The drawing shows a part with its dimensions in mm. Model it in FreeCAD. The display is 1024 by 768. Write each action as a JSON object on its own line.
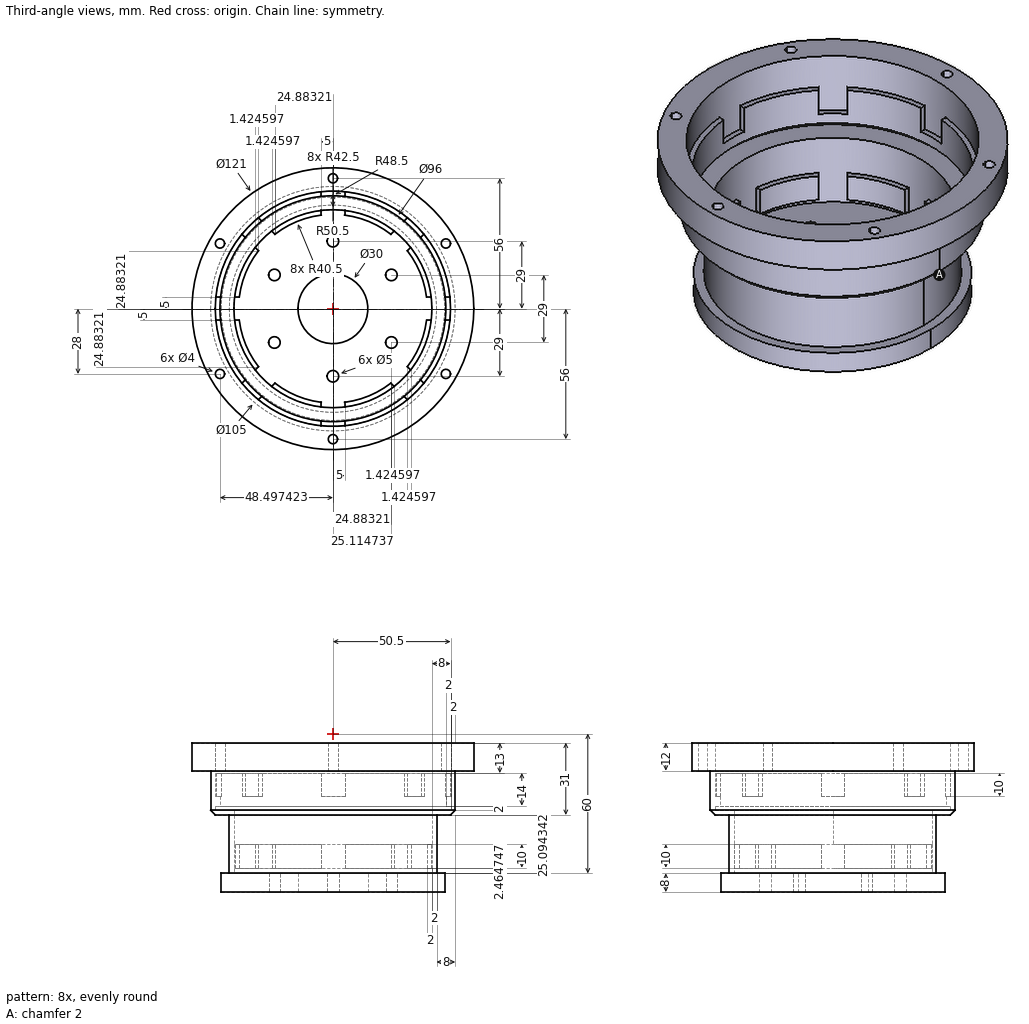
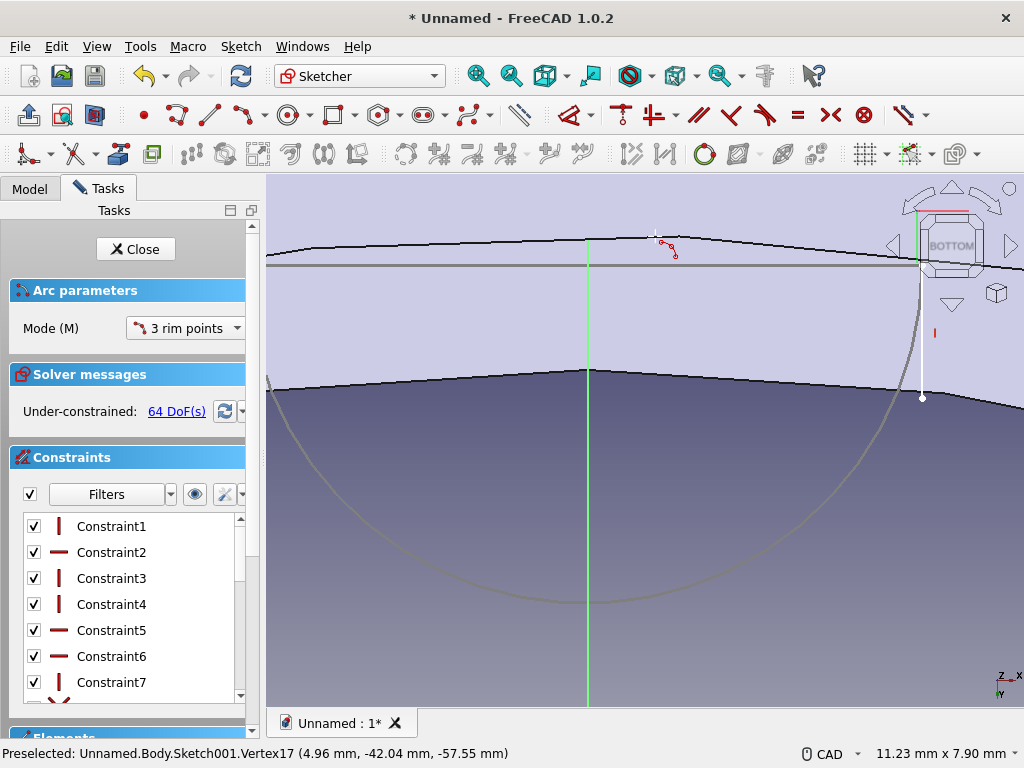
{"action": "left_click", "coordinate": [655, 236]}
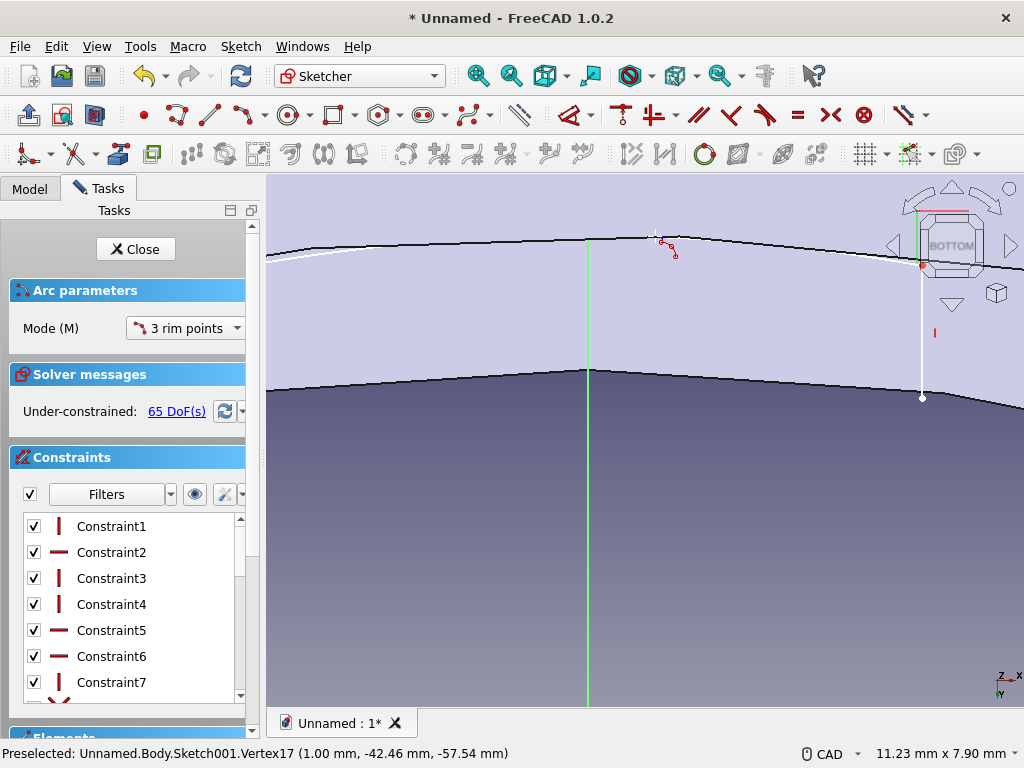
{"action": "scroll", "coordinate": [576, 268], "scroll_direction": "down", "scroll_amount": 14}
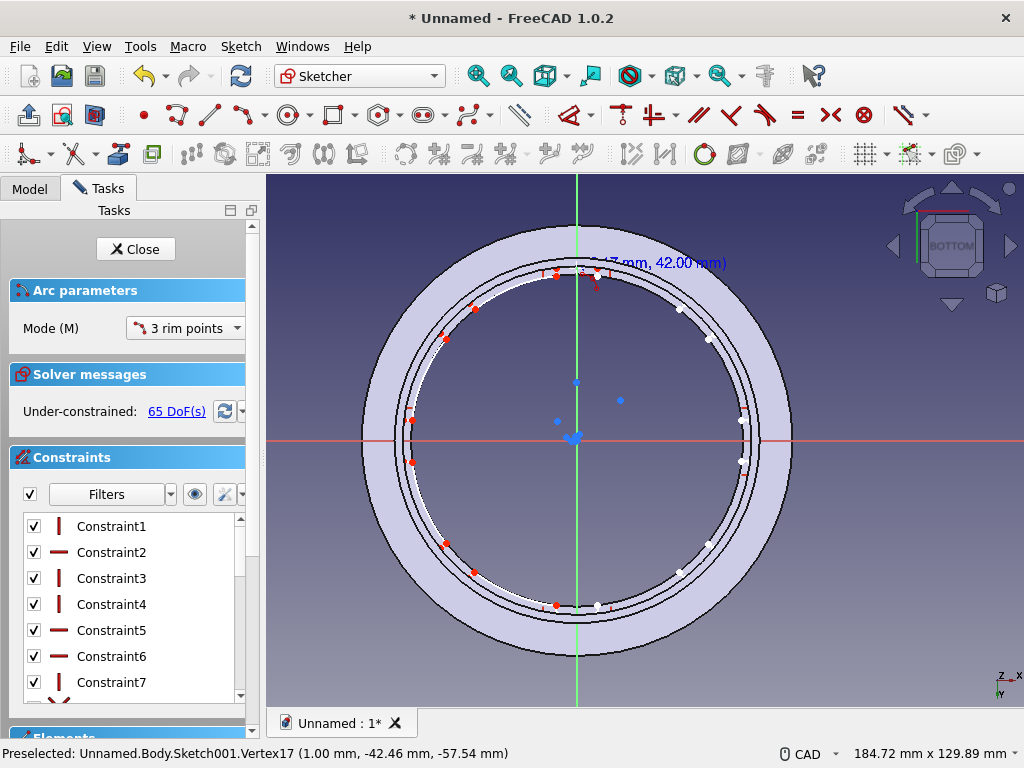
{"action": "scroll", "coordinate": [598, 276], "scroll_direction": "up", "scroll_amount": 7}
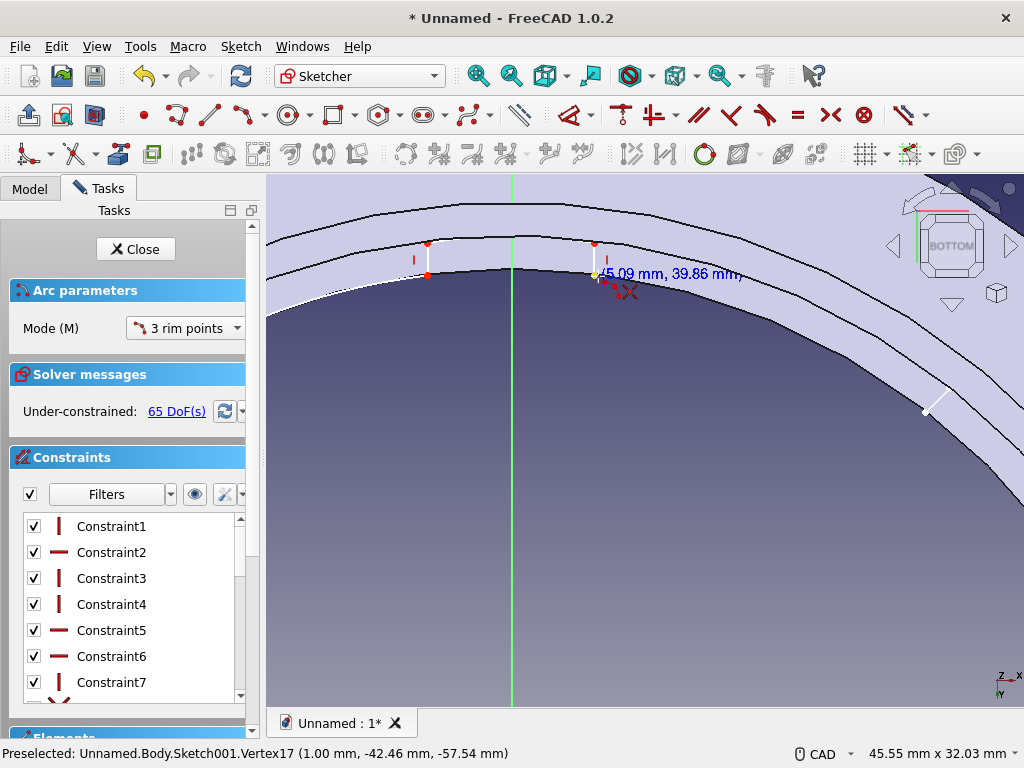
{"action": "left_click", "coordinate": [594, 276]}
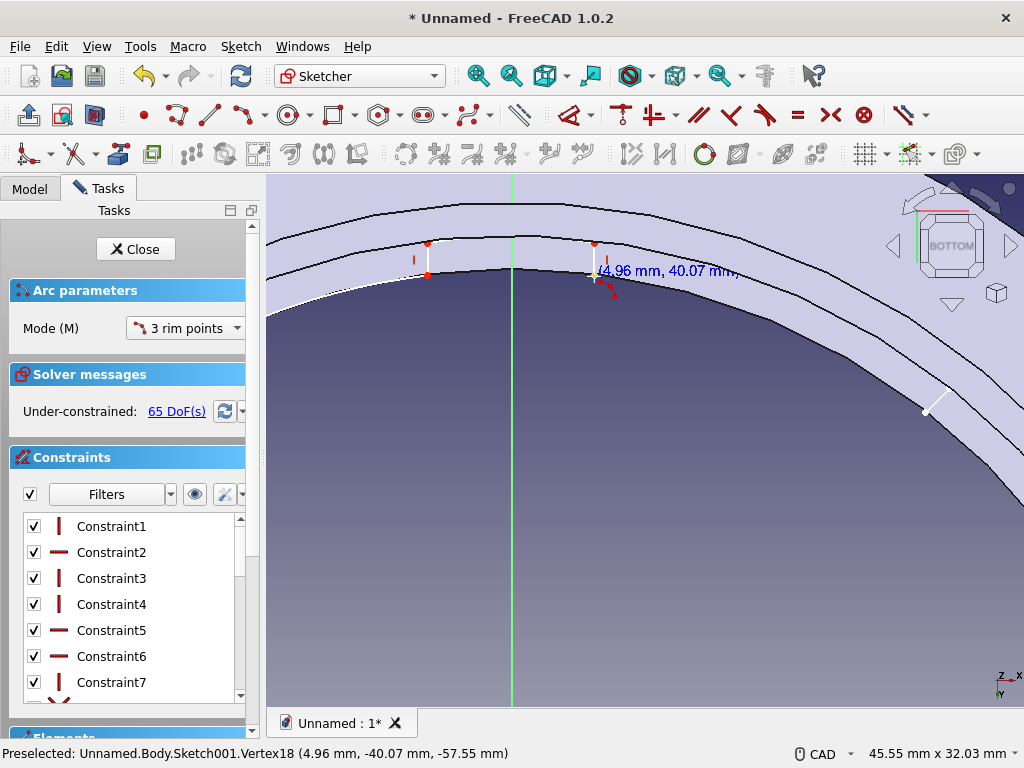
{"action": "scroll", "coordinate": [598, 276], "scroll_direction": "down", "scroll_amount": 7}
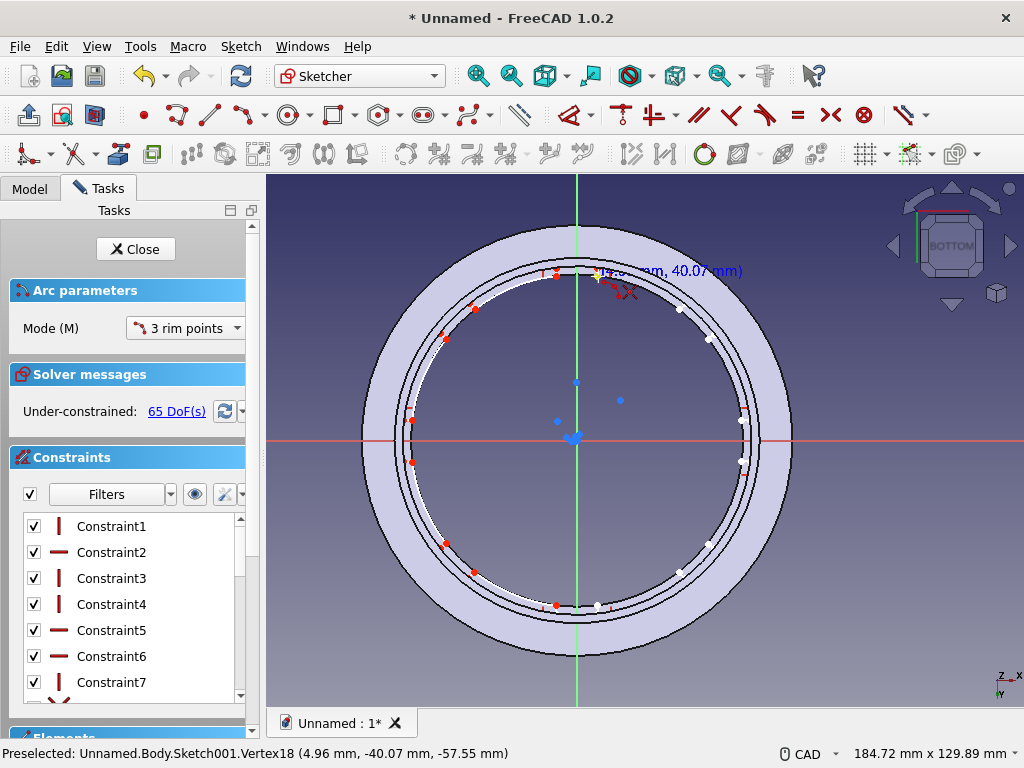
{"action": "scroll", "coordinate": [679, 309], "scroll_direction": "up", "scroll_amount": 7}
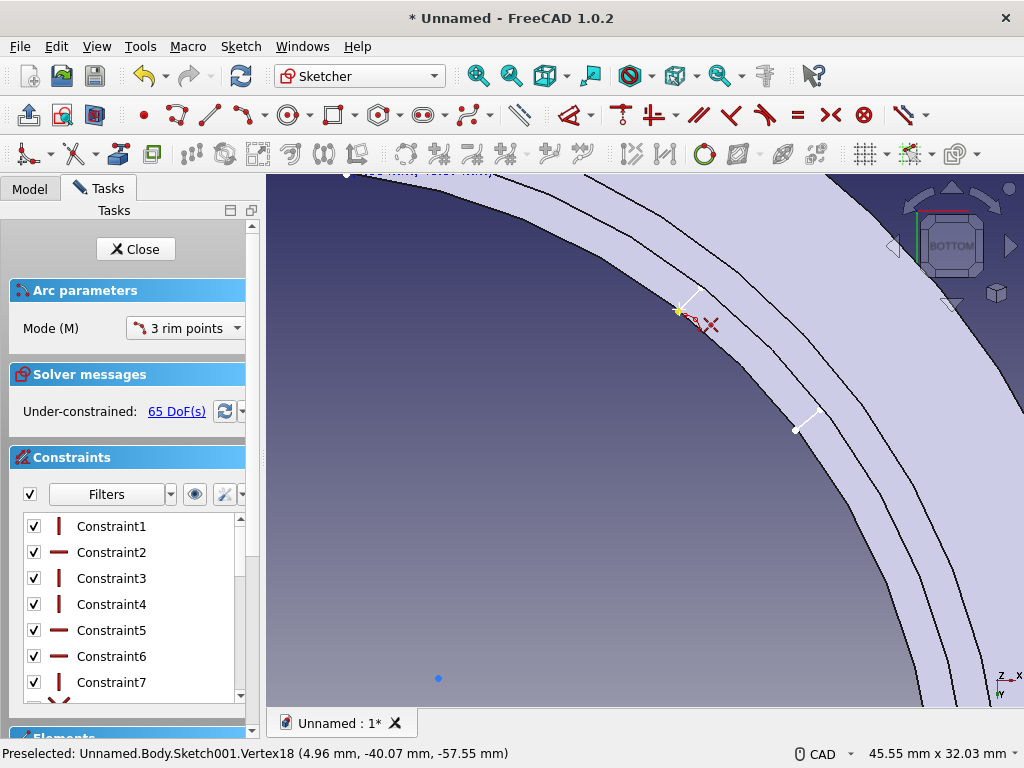
{"action": "left_click", "coordinate": [678, 312]}
{"action": "left_click", "coordinate": [522, 219]}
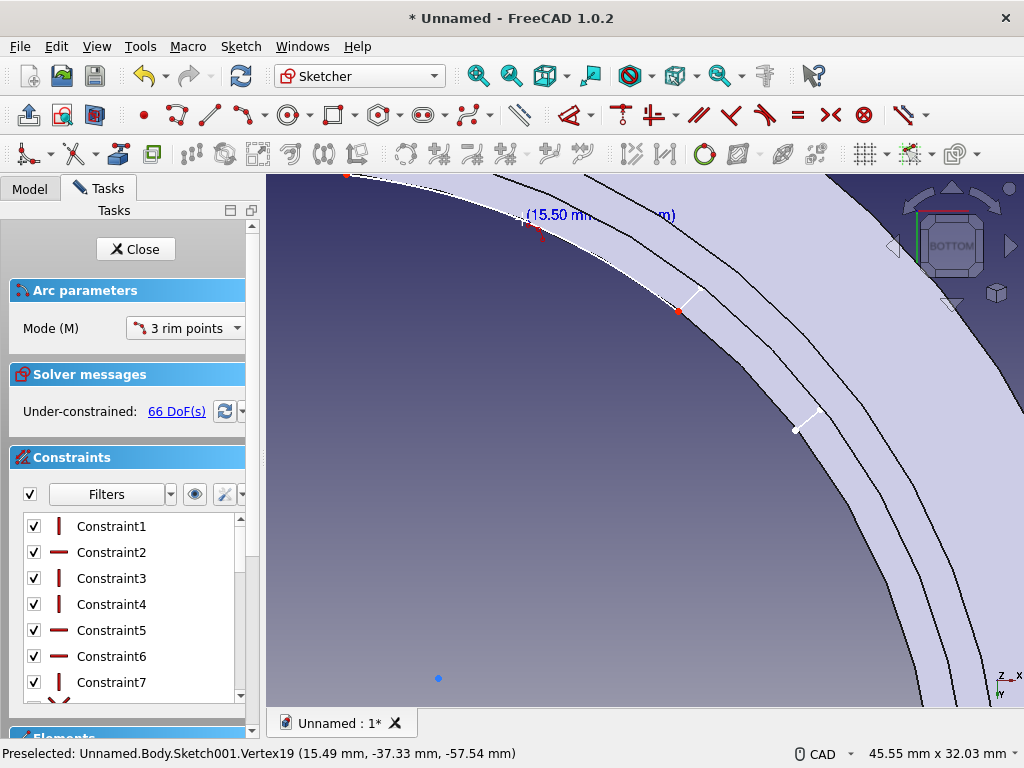
{"action": "left_click", "coordinate": [702, 288]}
{"action": "left_click", "coordinate": [821, 410]}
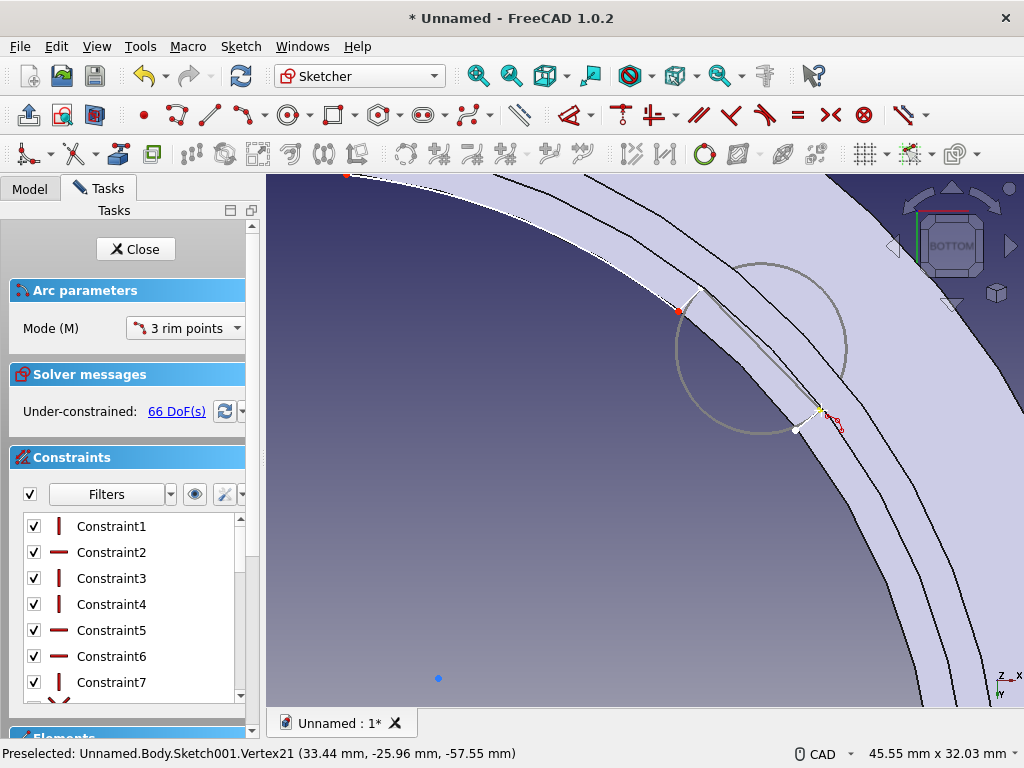
{"action": "scroll", "coordinate": [764, 342], "scroll_direction": "up", "scroll_amount": 6}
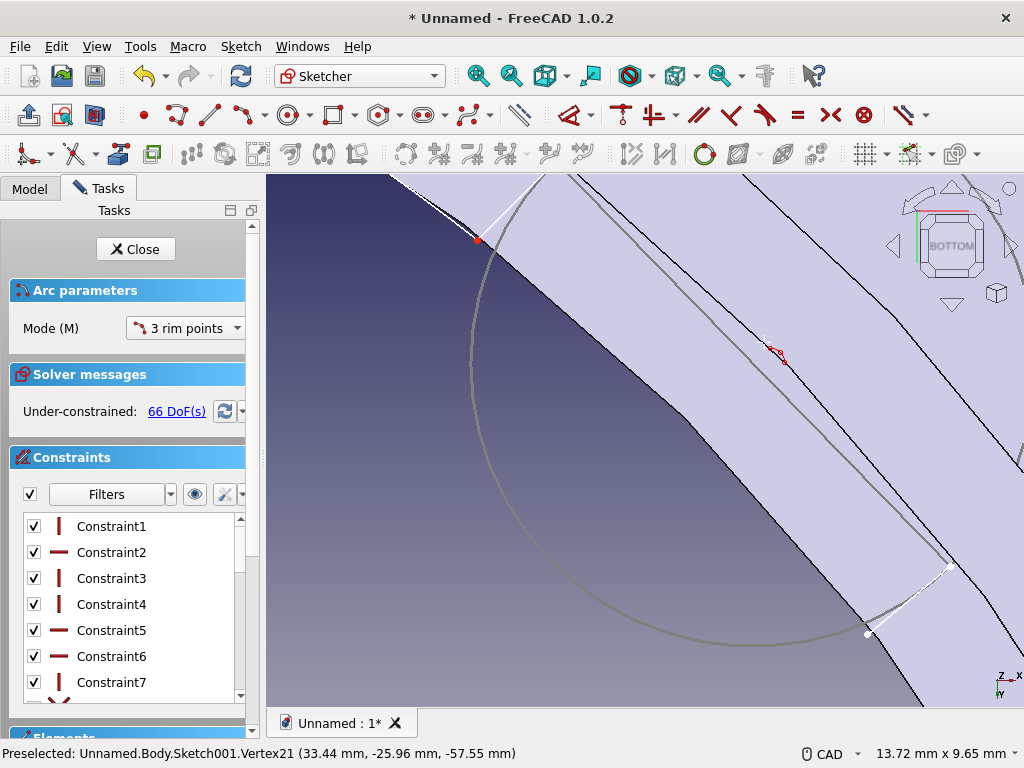
{"action": "left_click", "coordinate": [763, 340]}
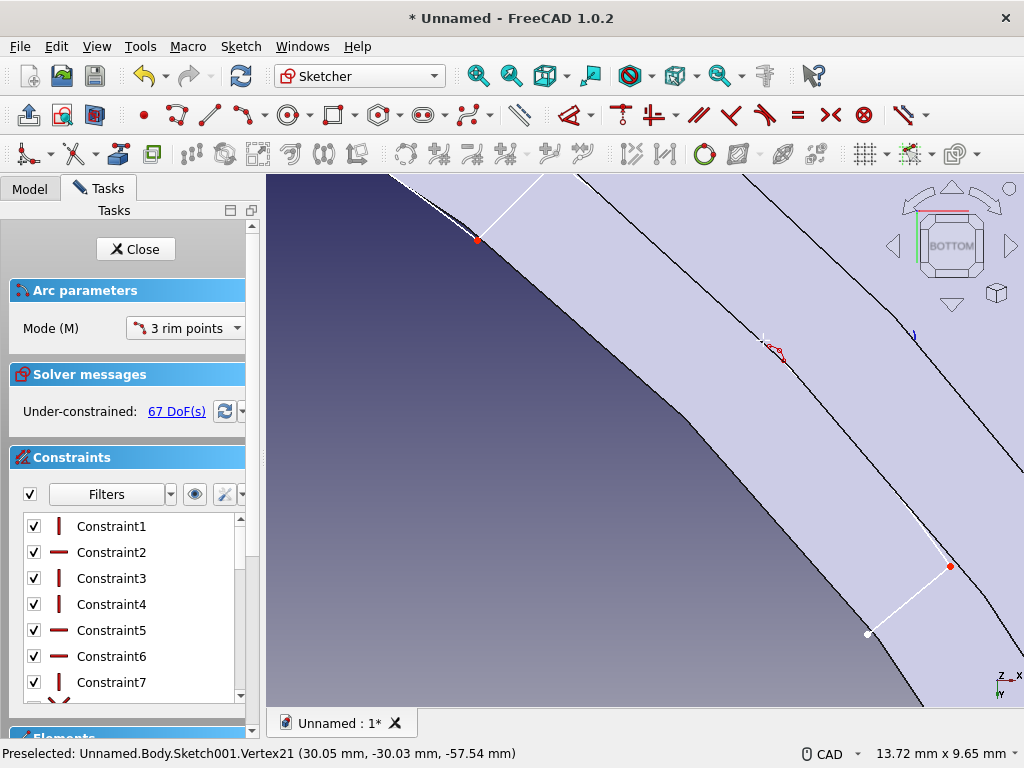
{"action": "scroll", "coordinate": [695, 315], "scroll_direction": "down", "scroll_amount": 13}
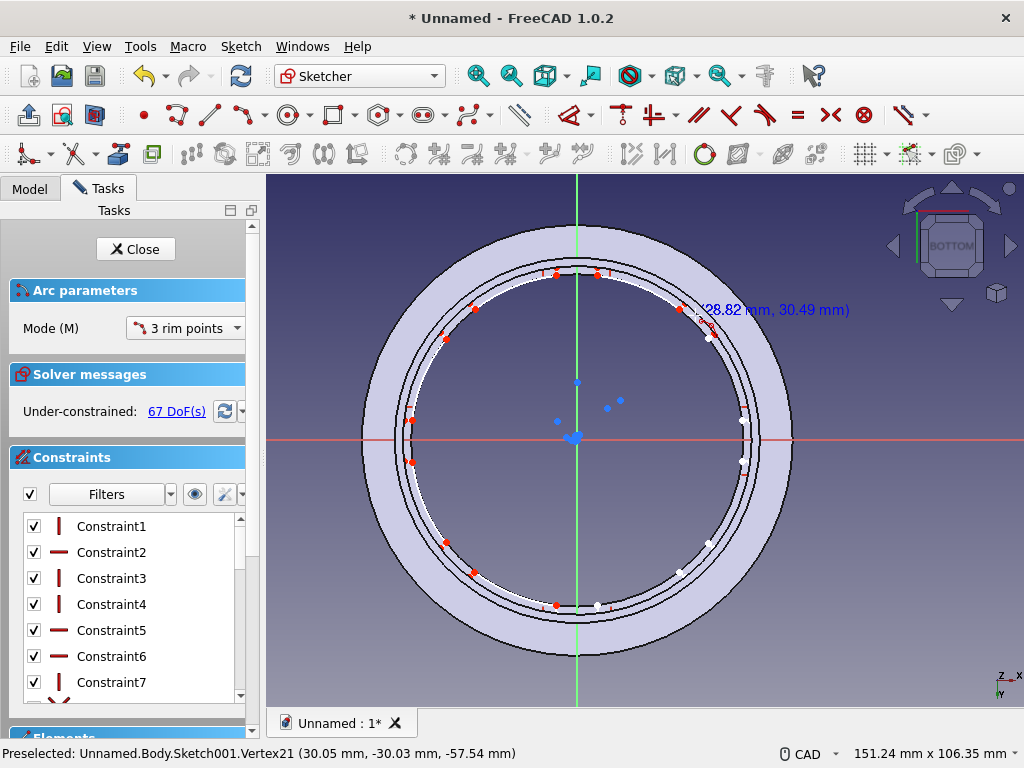
{"action": "scroll", "coordinate": [708, 338], "scroll_direction": "up", "scroll_amount": 7}